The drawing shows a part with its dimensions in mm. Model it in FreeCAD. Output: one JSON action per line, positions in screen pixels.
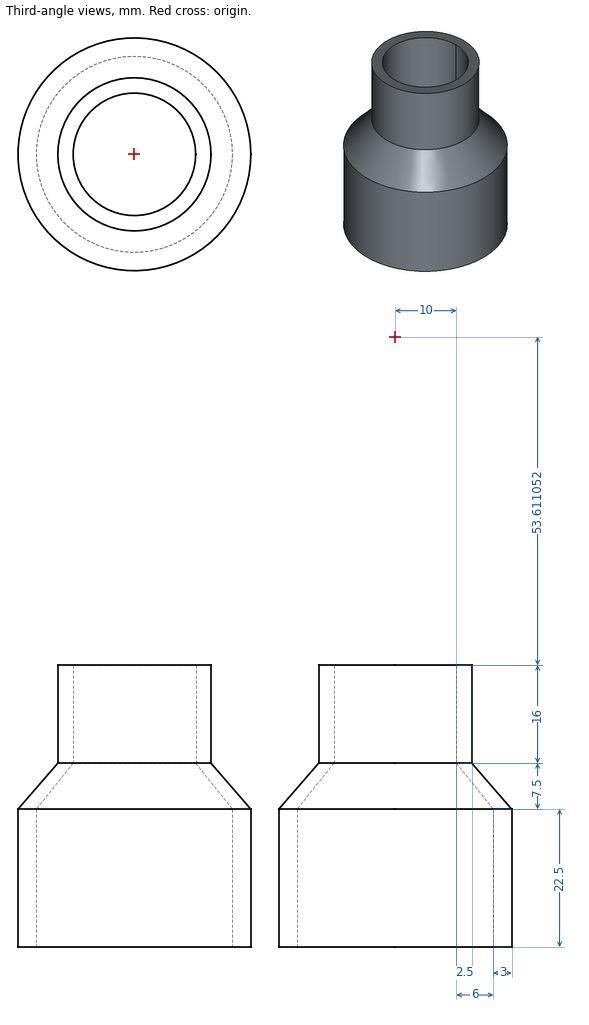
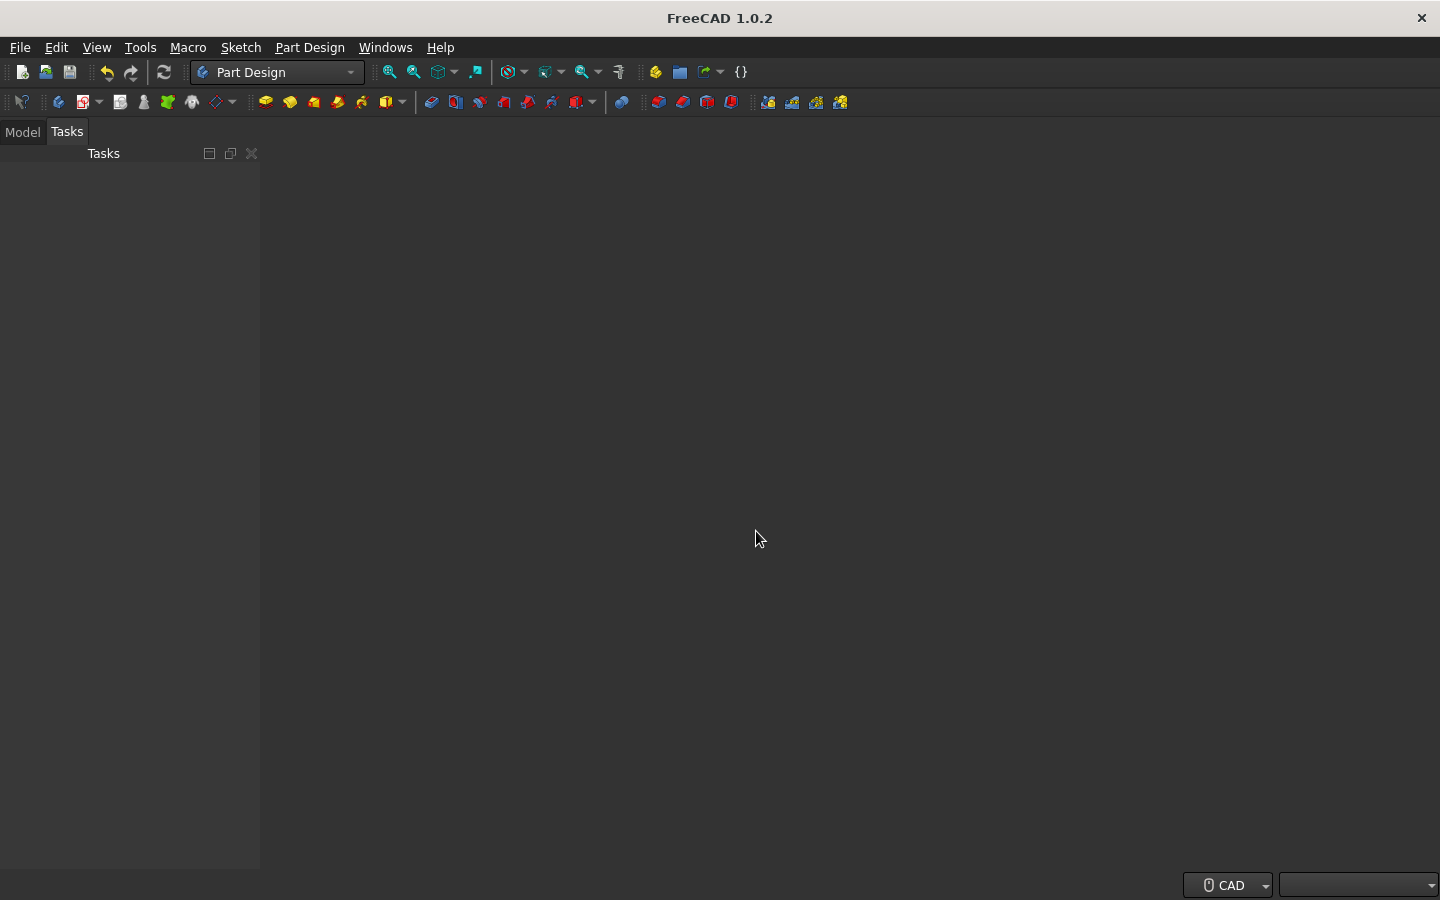
{"action": "key", "text": "ctrl+n"}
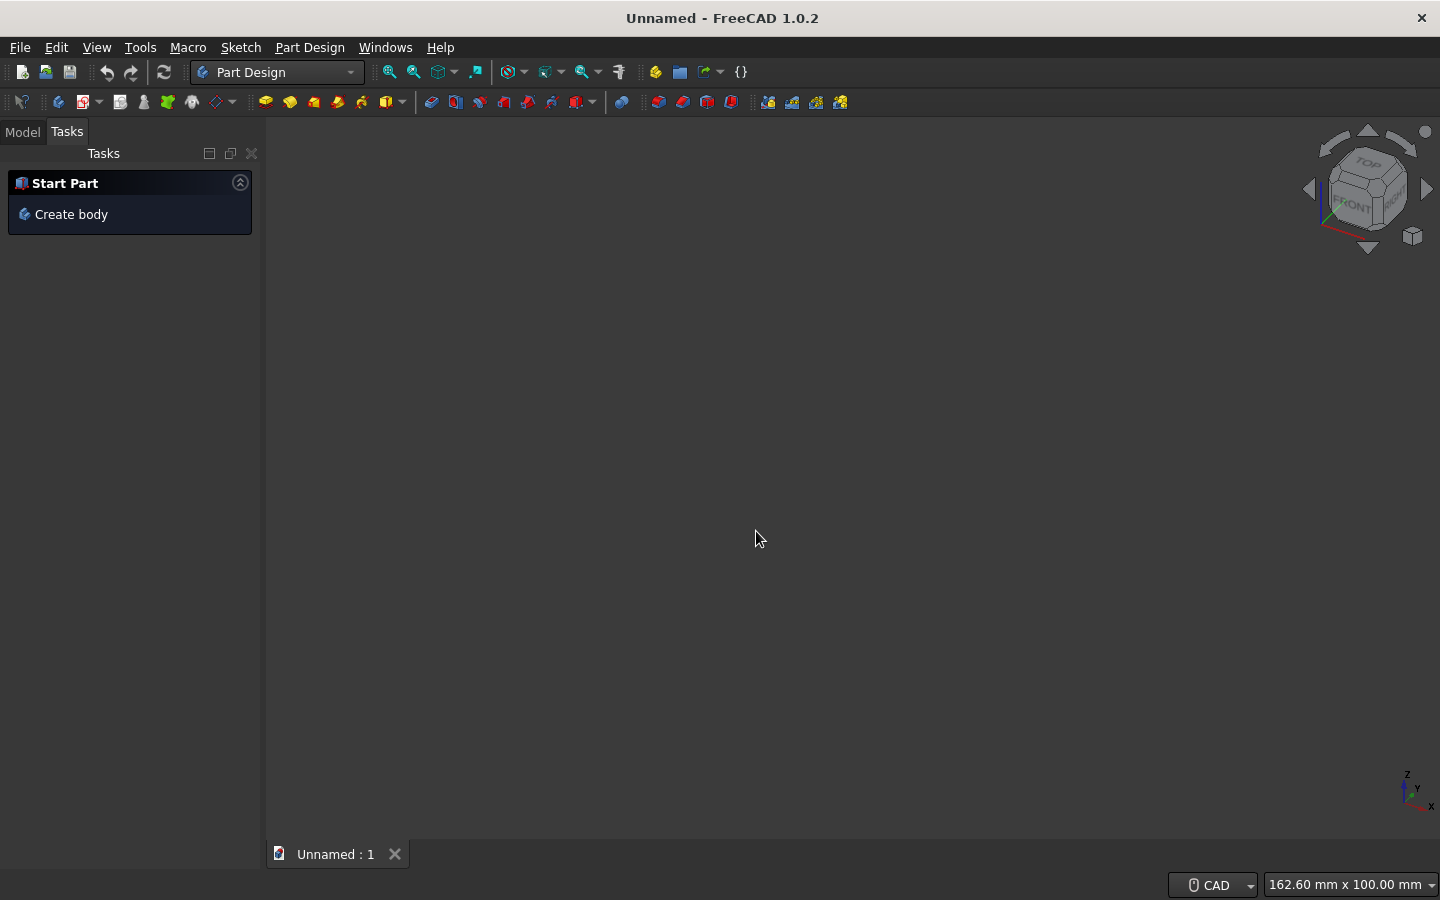
{"action": "left_click", "coordinate": [84, 102]}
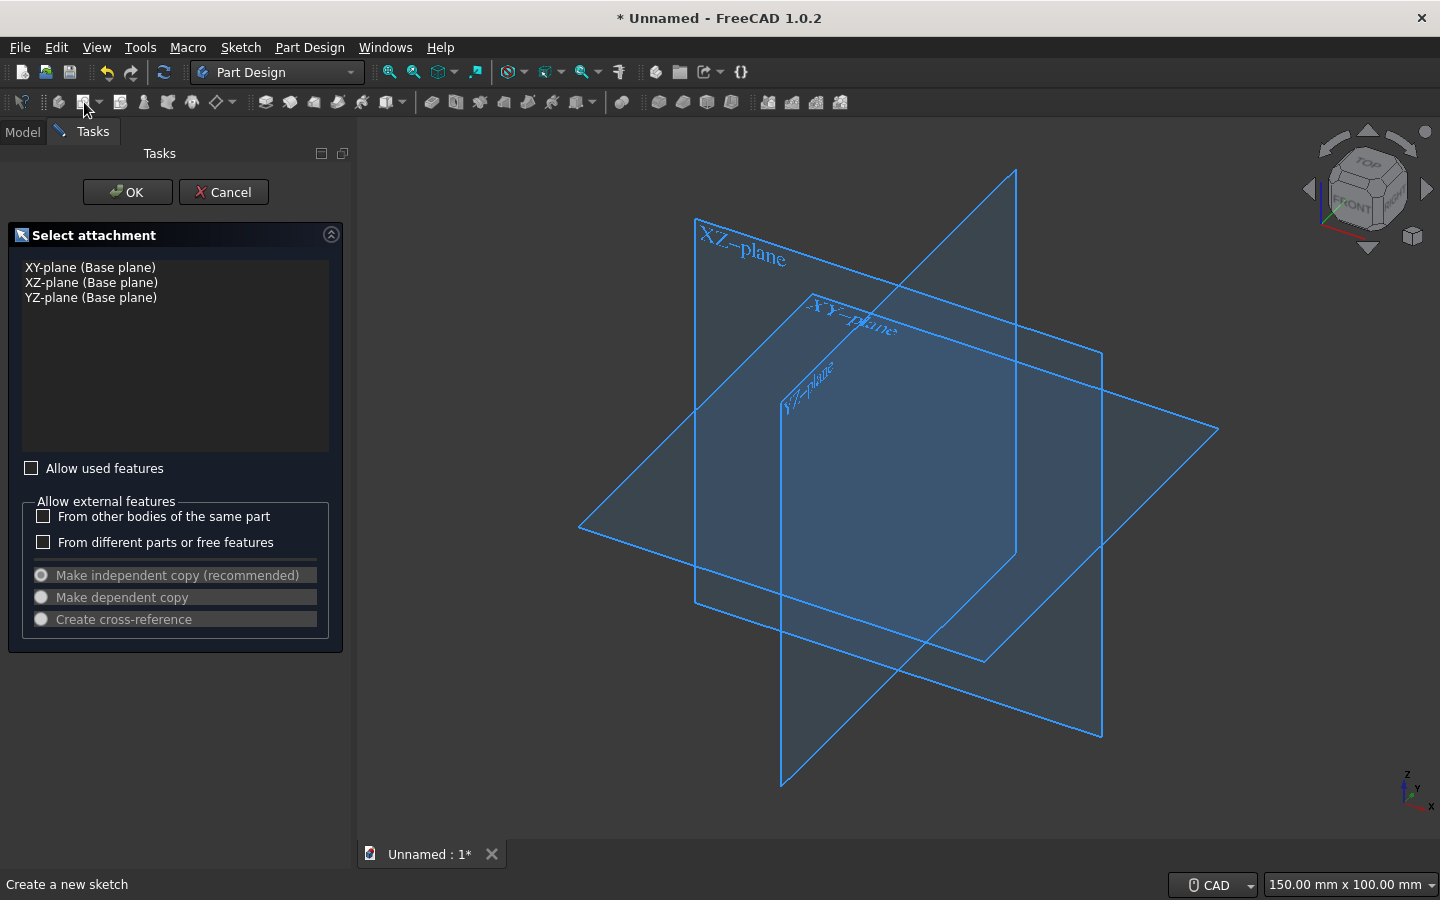
{"action": "left_click", "coordinate": [82, 298]}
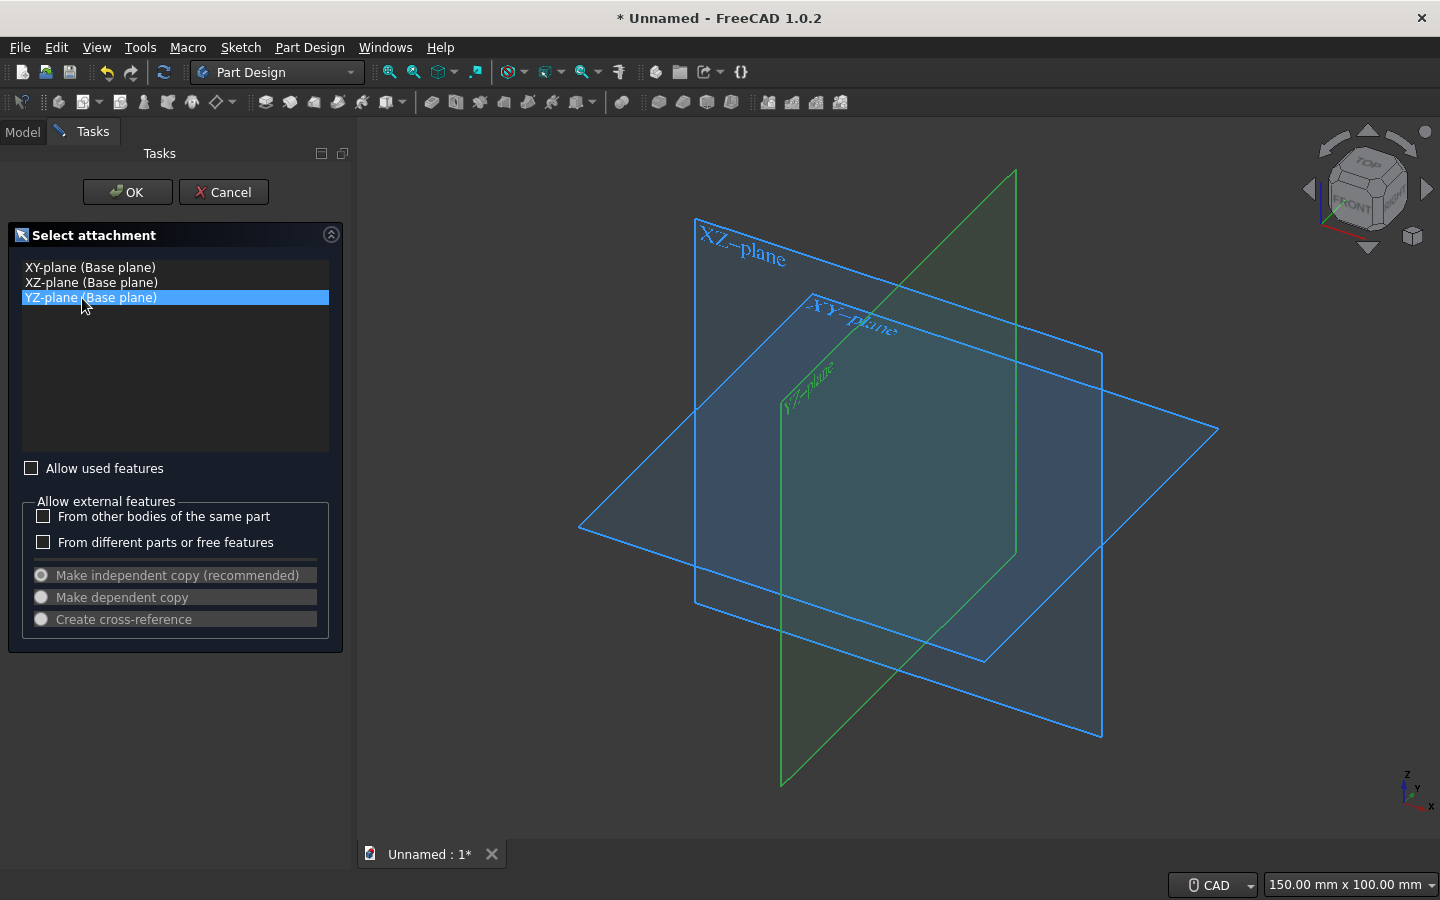
{"action": "left_click", "coordinate": [128, 192]}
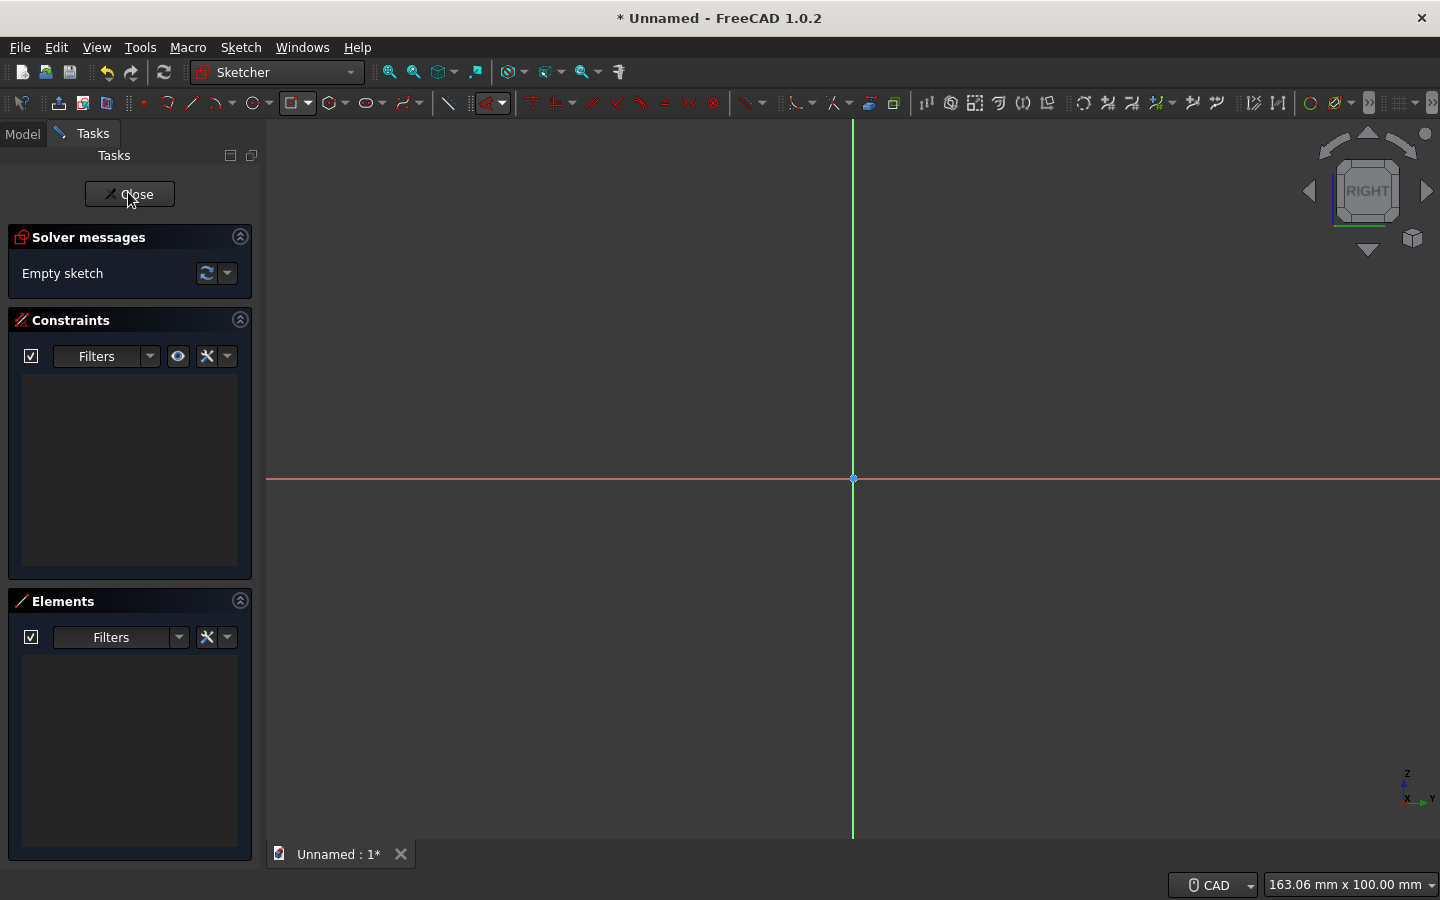
{"action": "scroll", "coordinate": [618, 147], "scroll_direction": "down", "scroll_amount": 3}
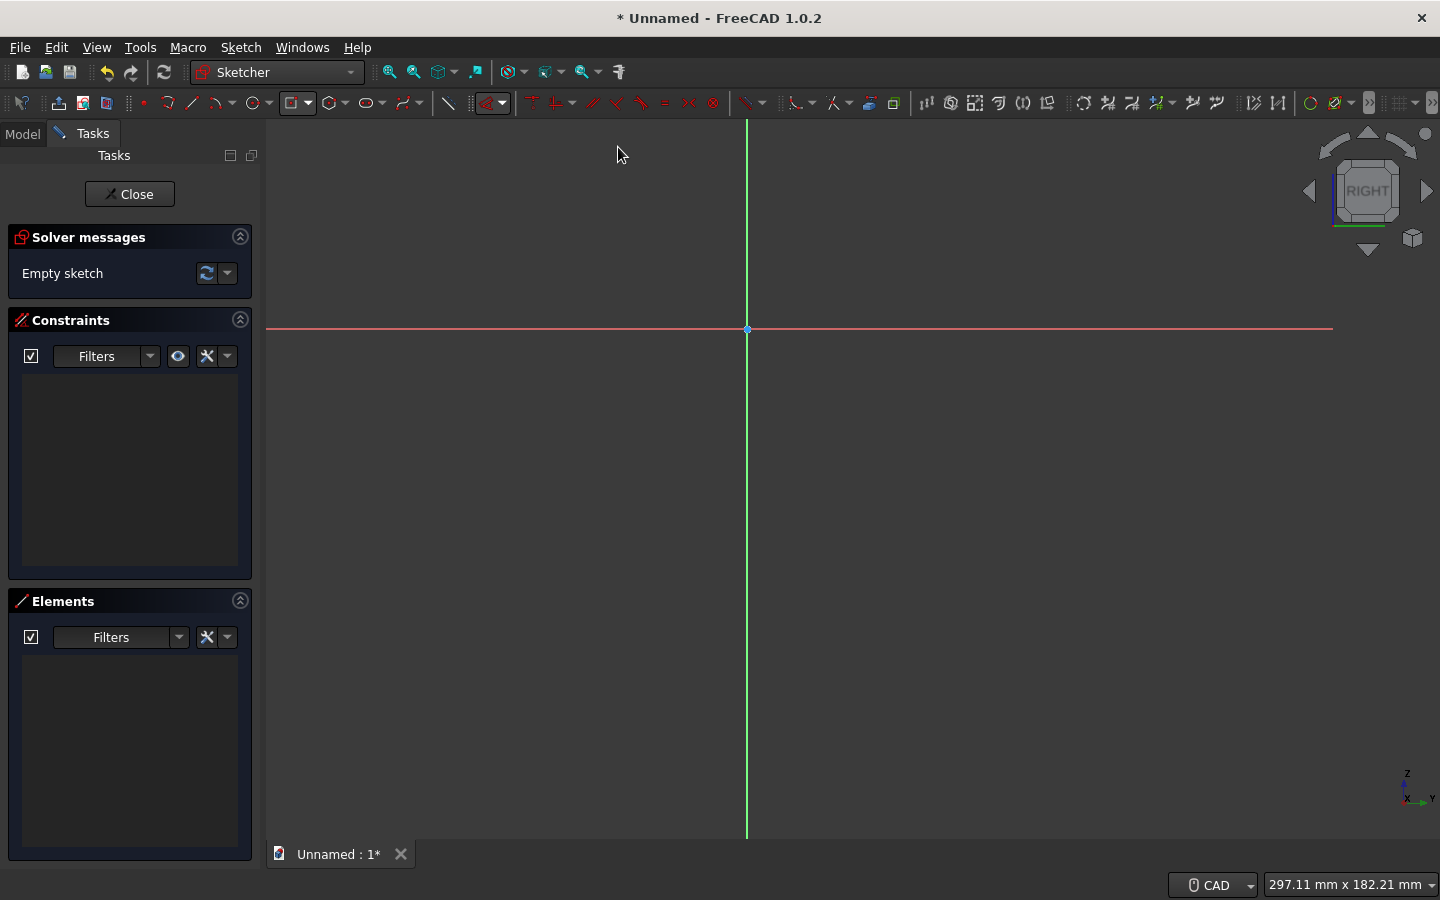
{"action": "left_click", "coordinate": [168, 104]}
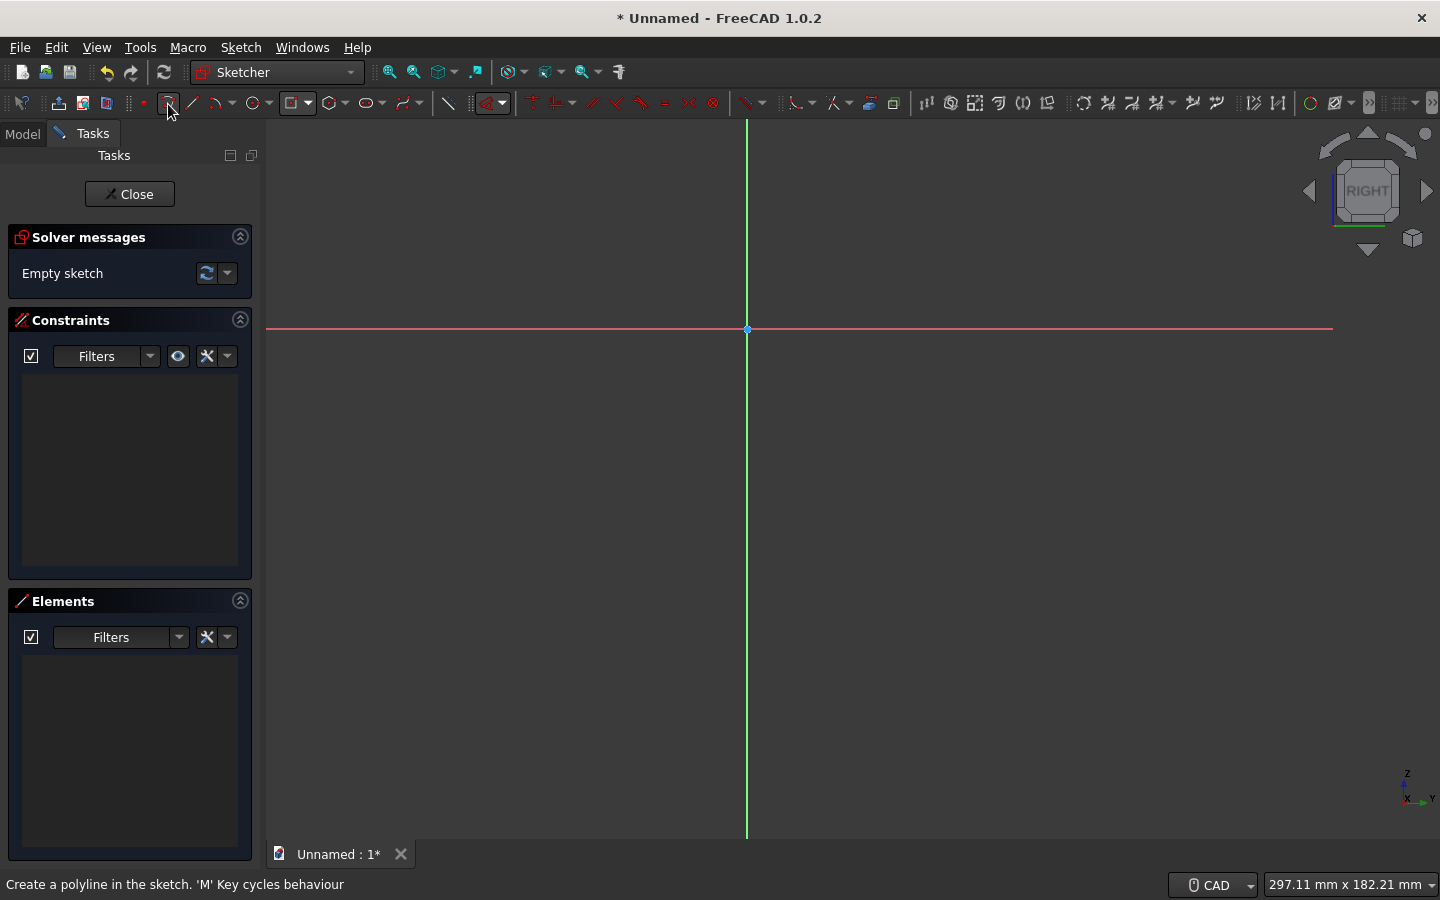
{"action": "left_click", "coordinate": [787, 541]}
{"action": "left_click", "coordinate": [787, 604]}
{"action": "left_click", "coordinate": [810, 634]}
{"action": "left_click", "coordinate": [810, 723]}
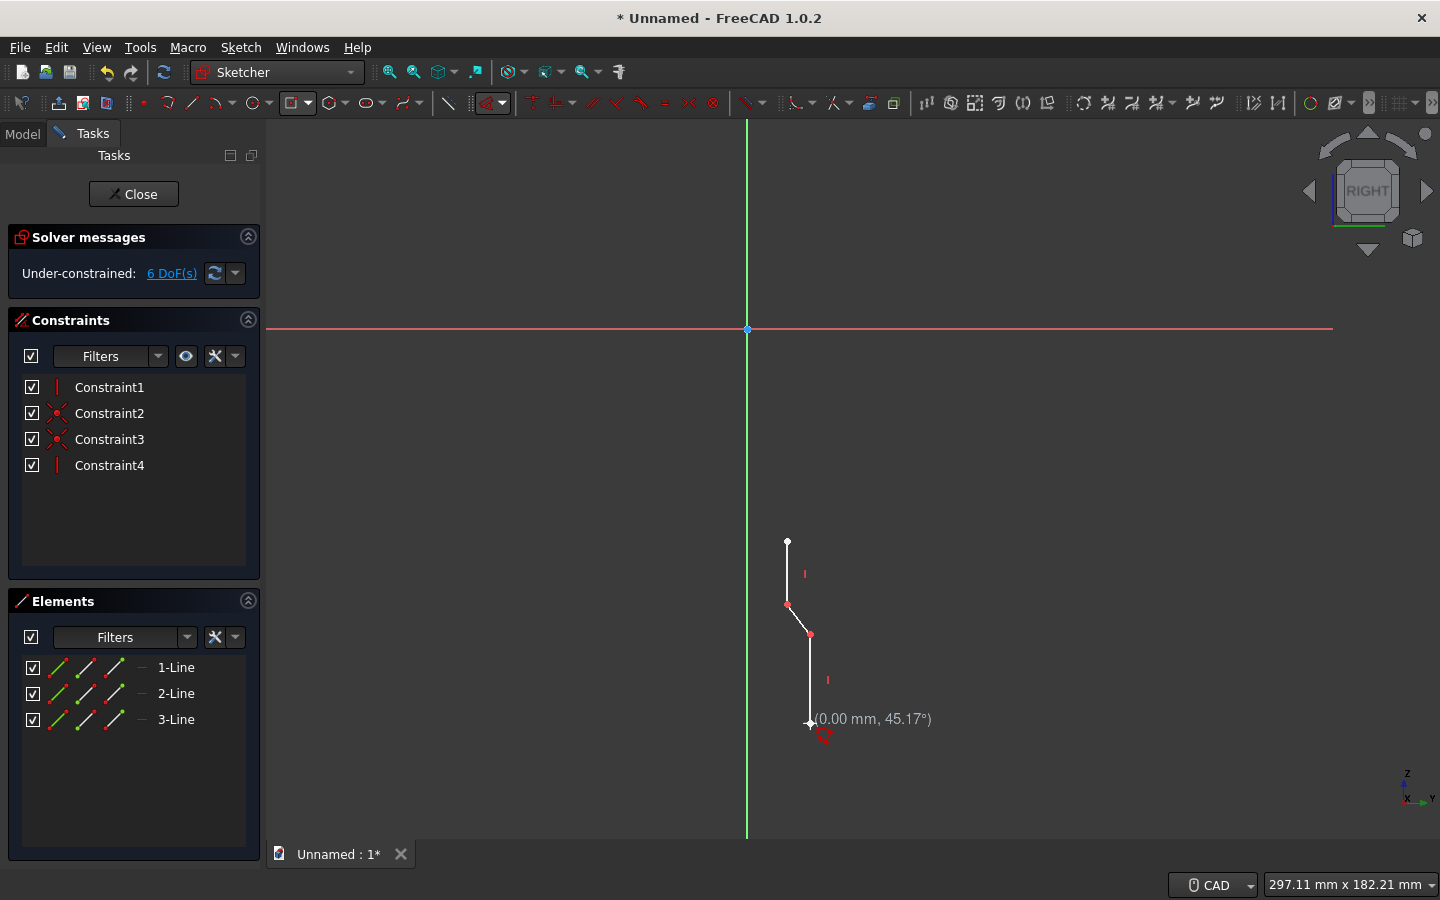
{"action": "scroll", "coordinate": [822, 723], "scroll_direction": "up", "scroll_amount": 2}